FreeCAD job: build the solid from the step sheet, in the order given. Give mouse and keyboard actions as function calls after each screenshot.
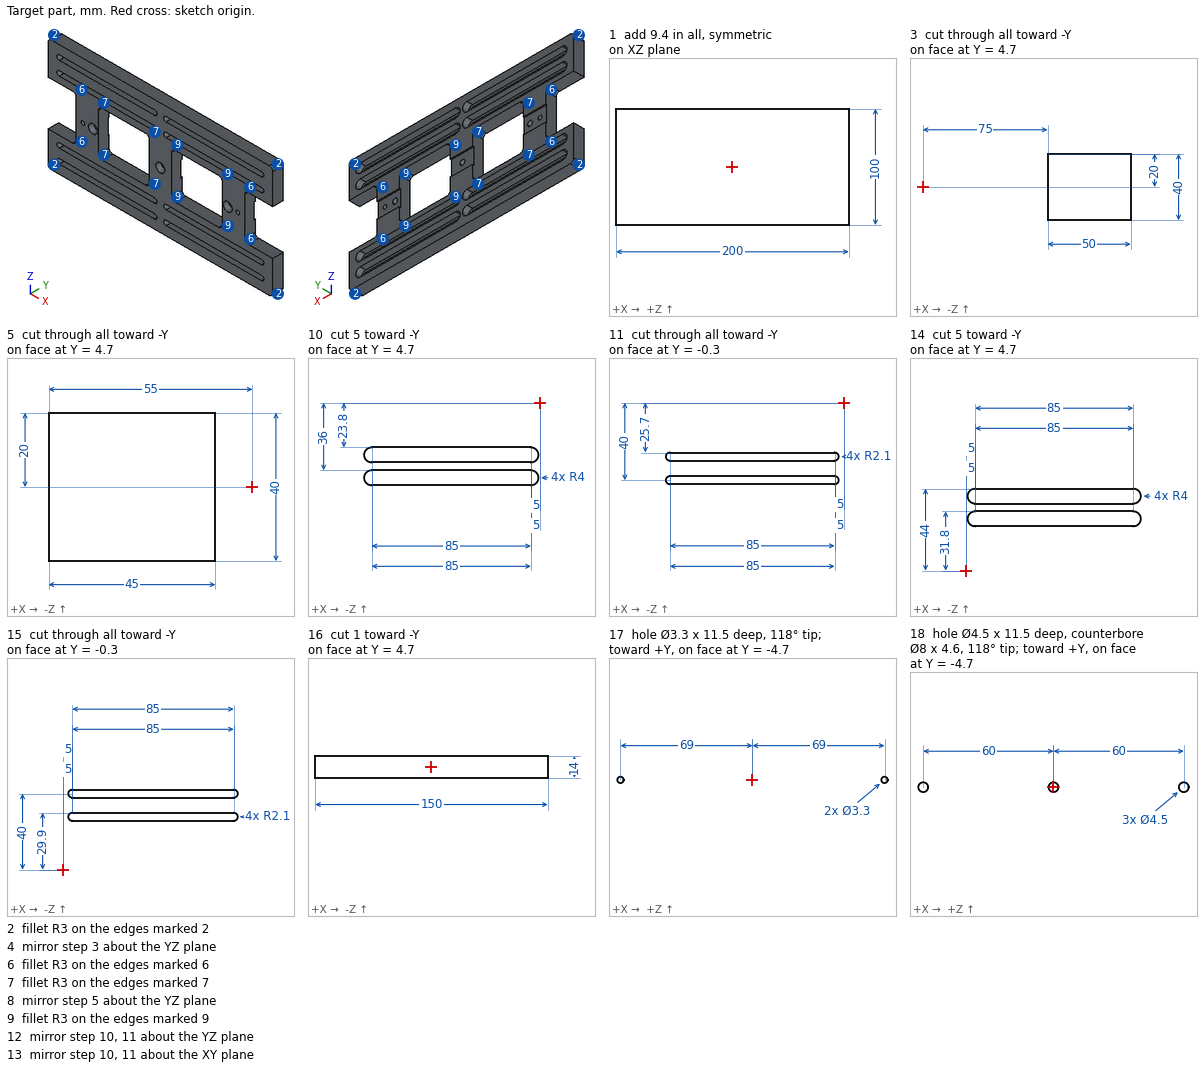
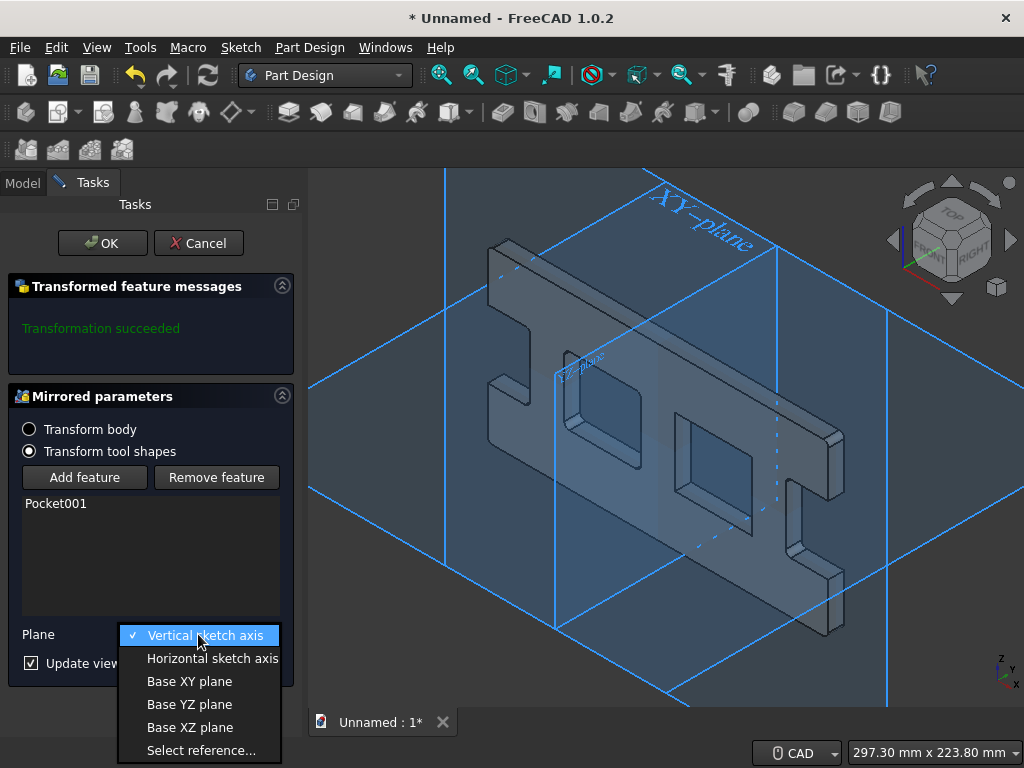
click(198, 704)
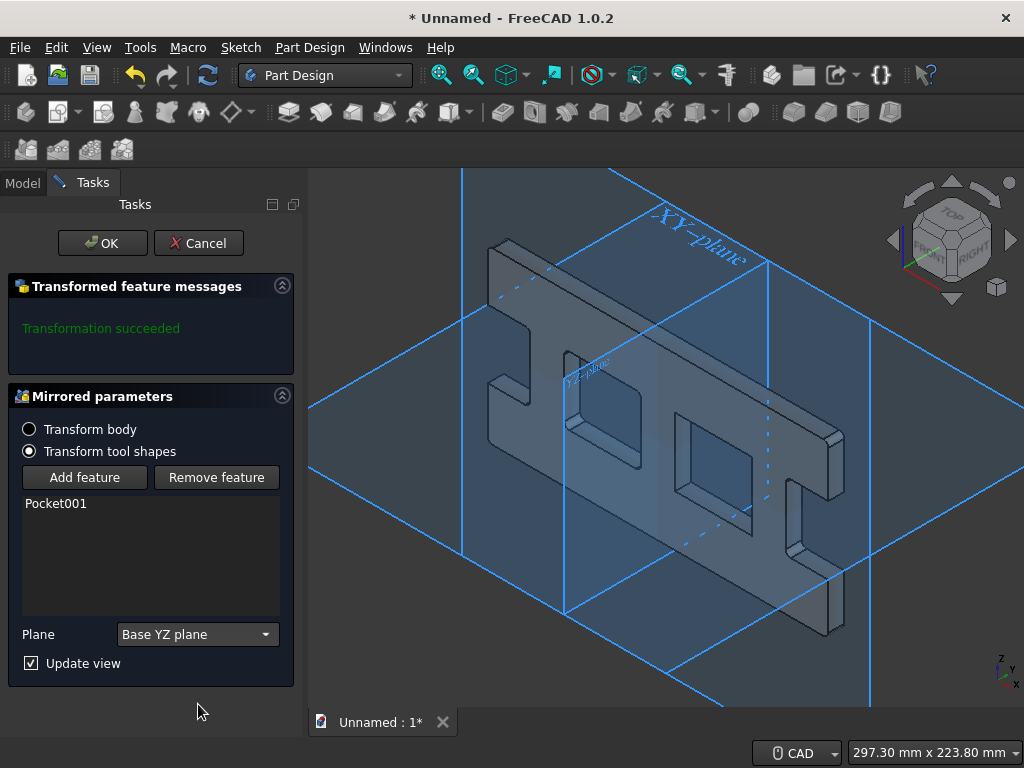
click(103, 243)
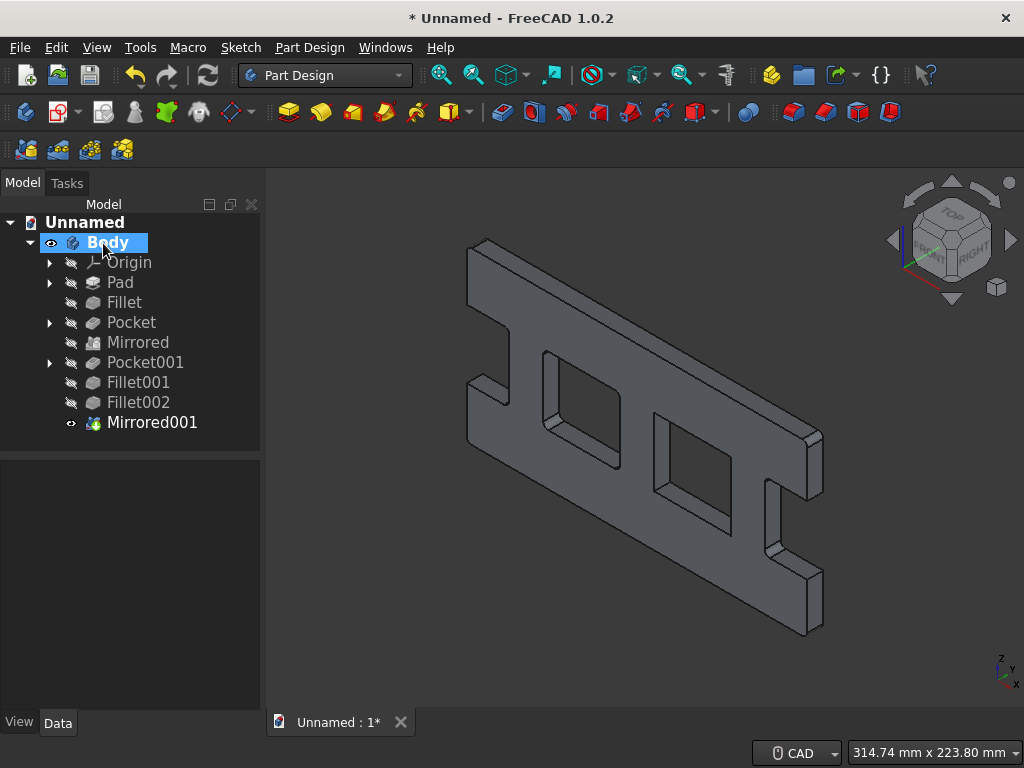
key(2)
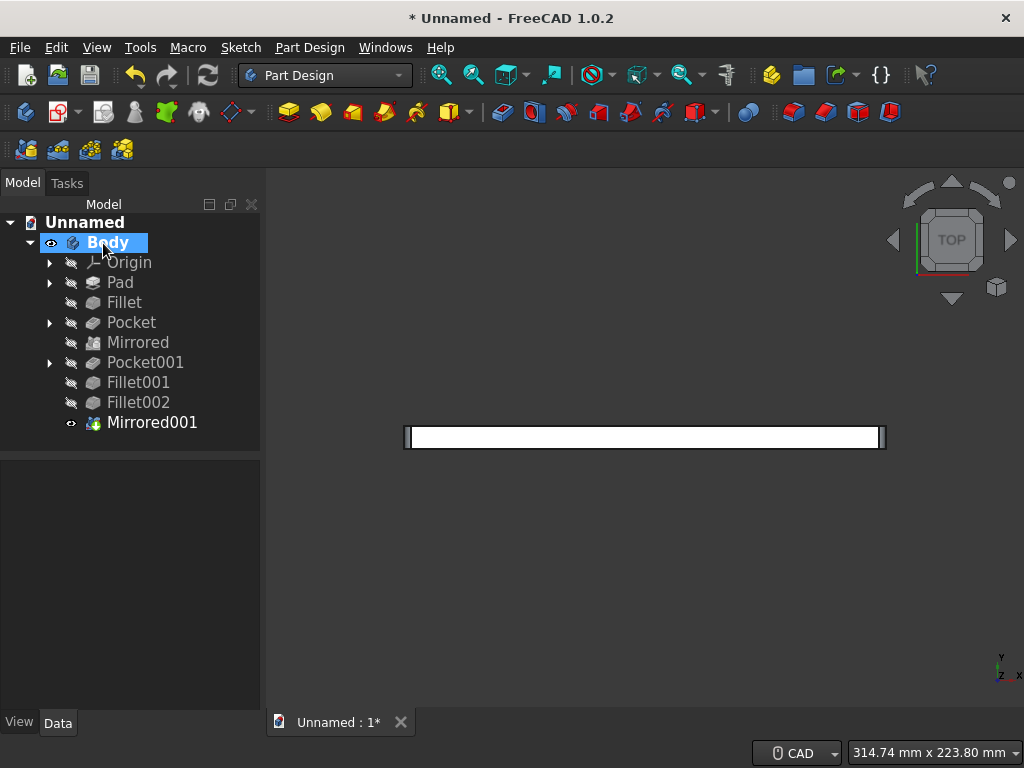
key(0)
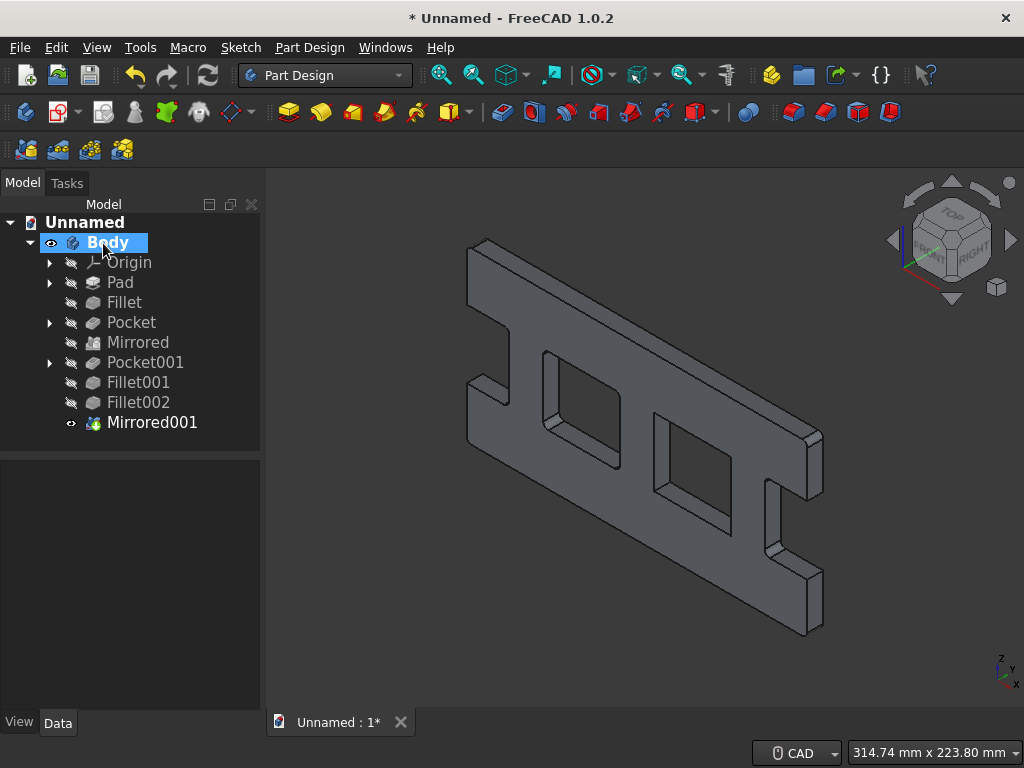
key(1)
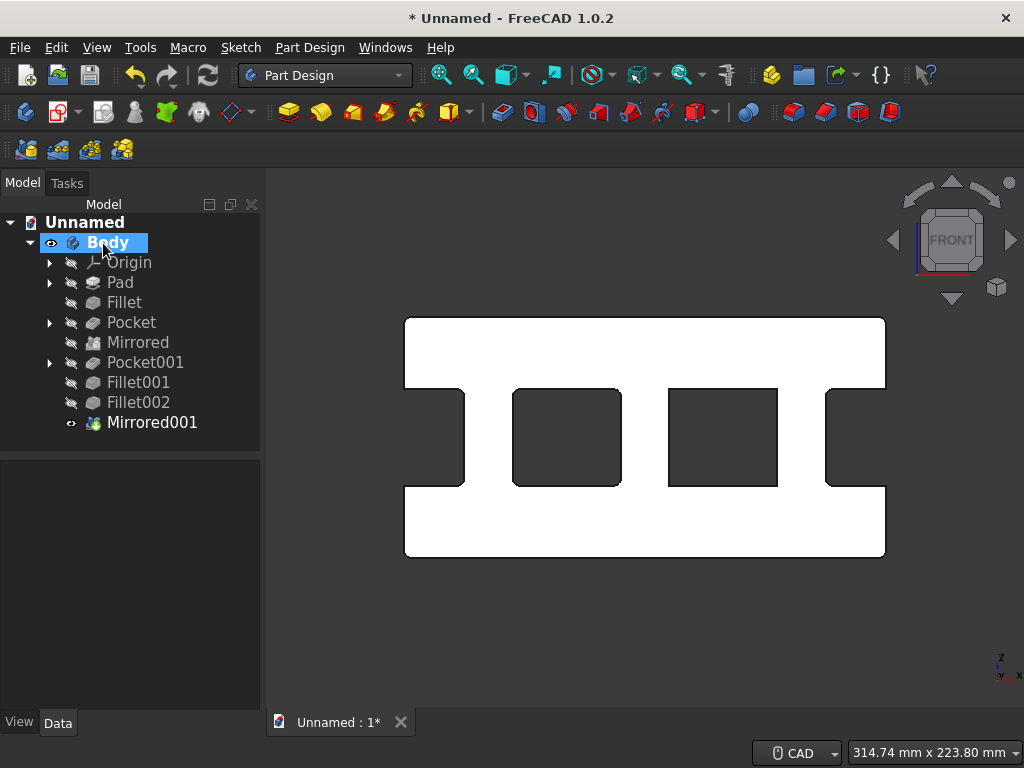
key(3)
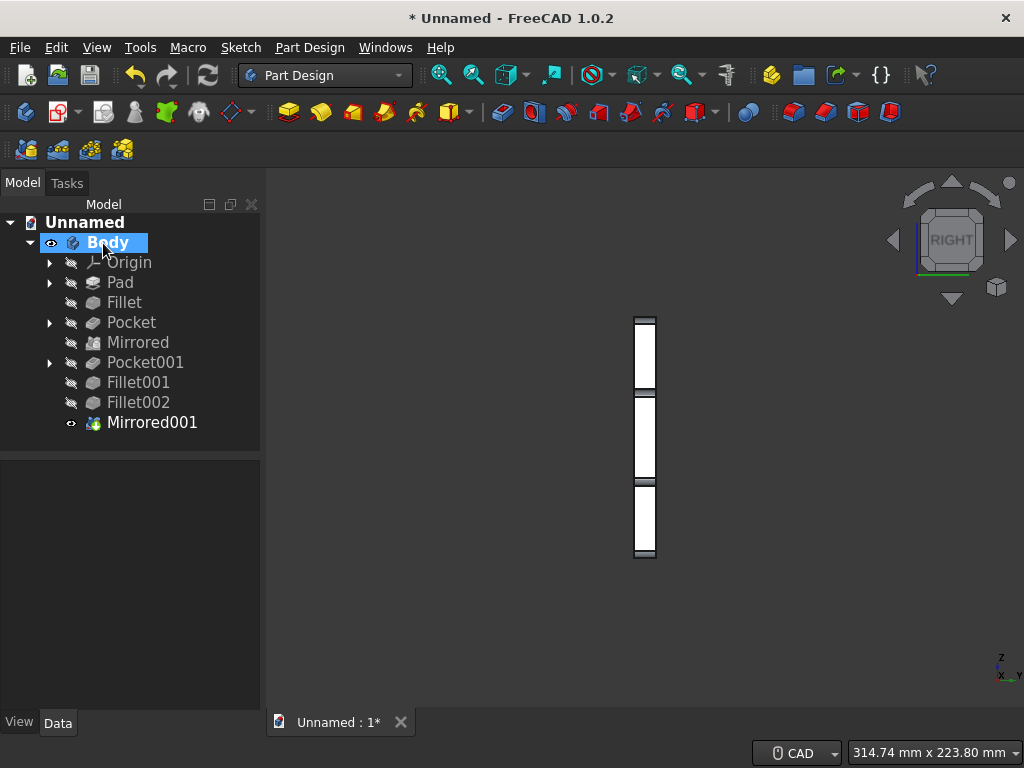
key(v)
key(f)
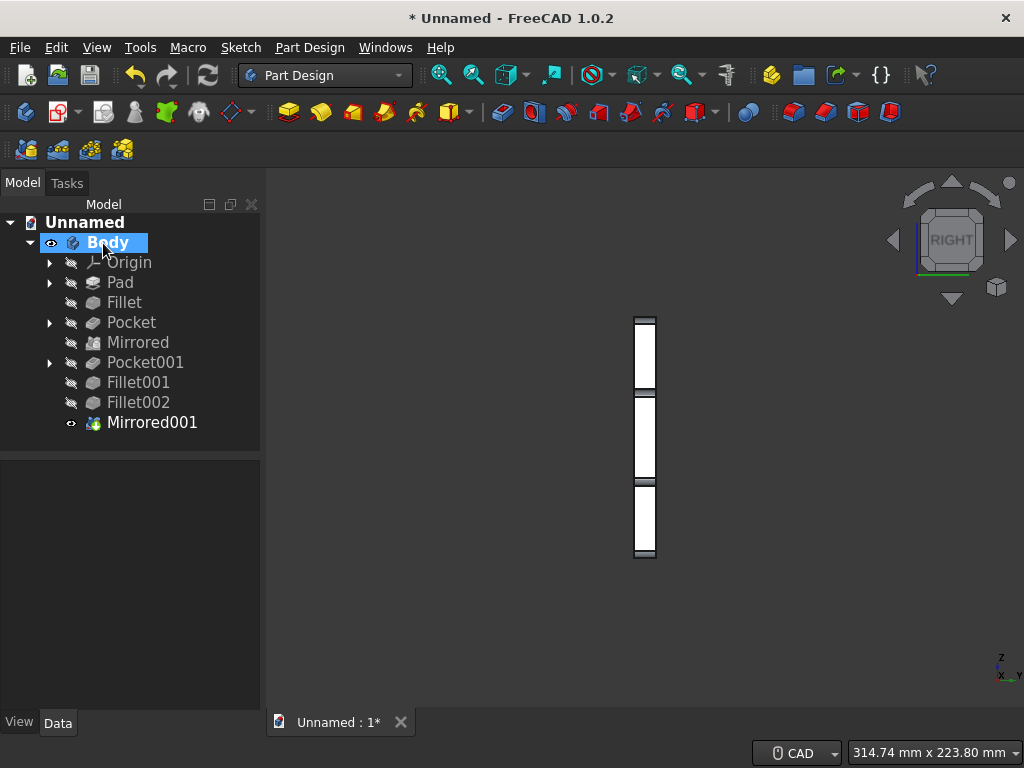
key(5)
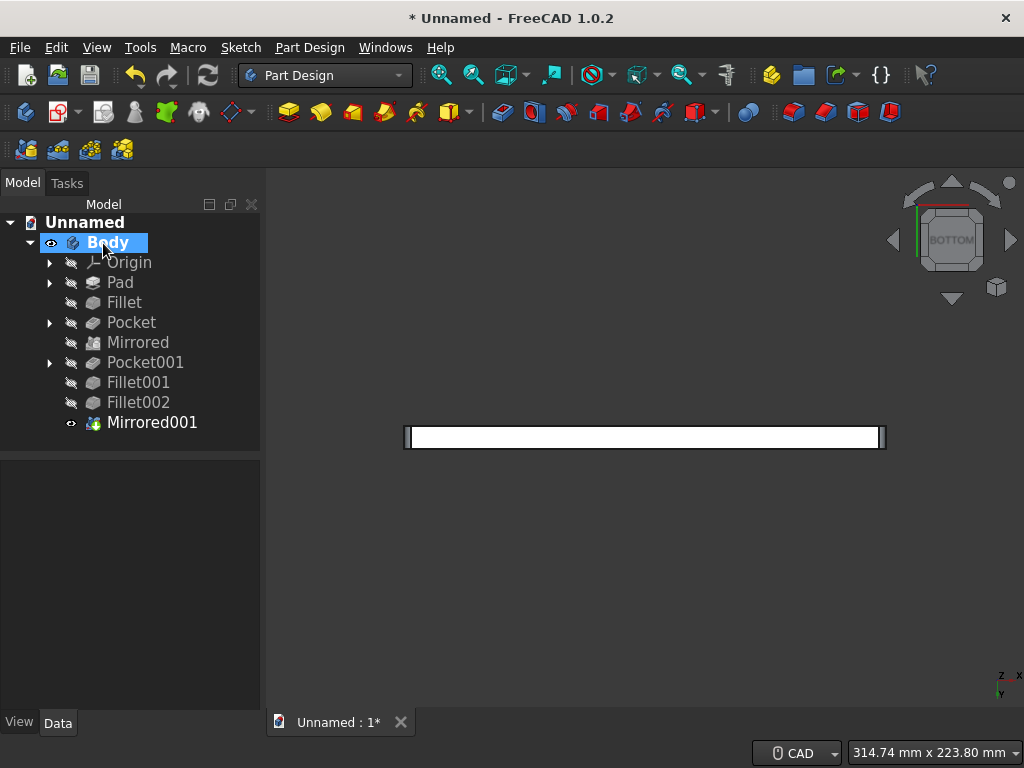
key(4)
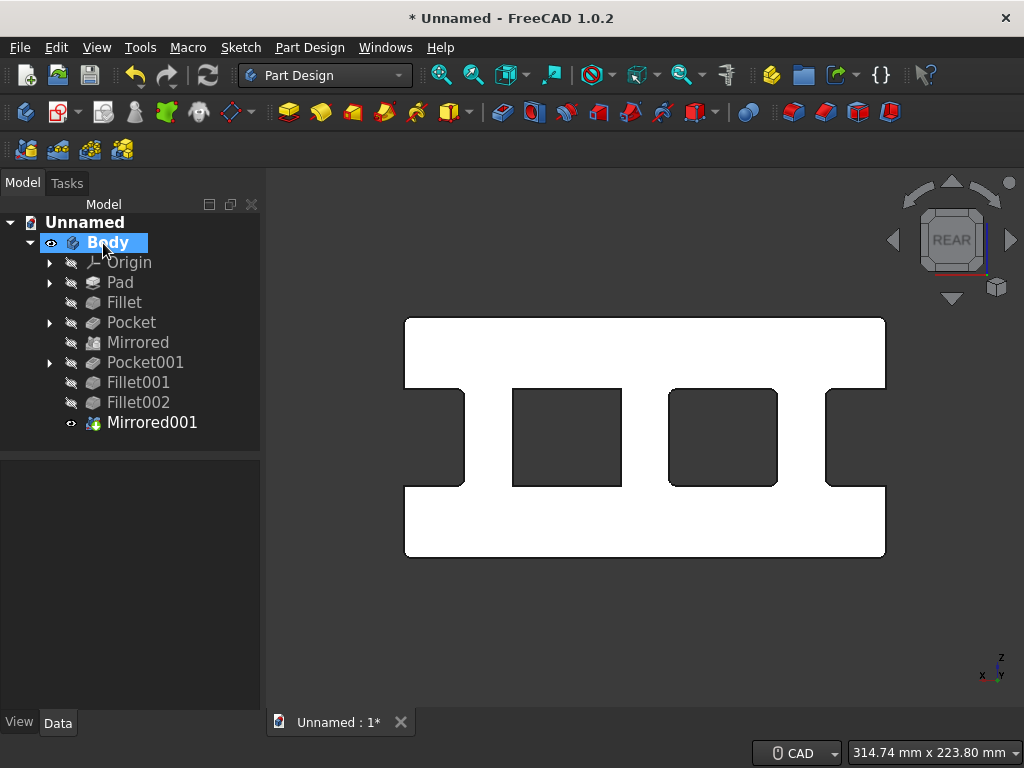
key(6)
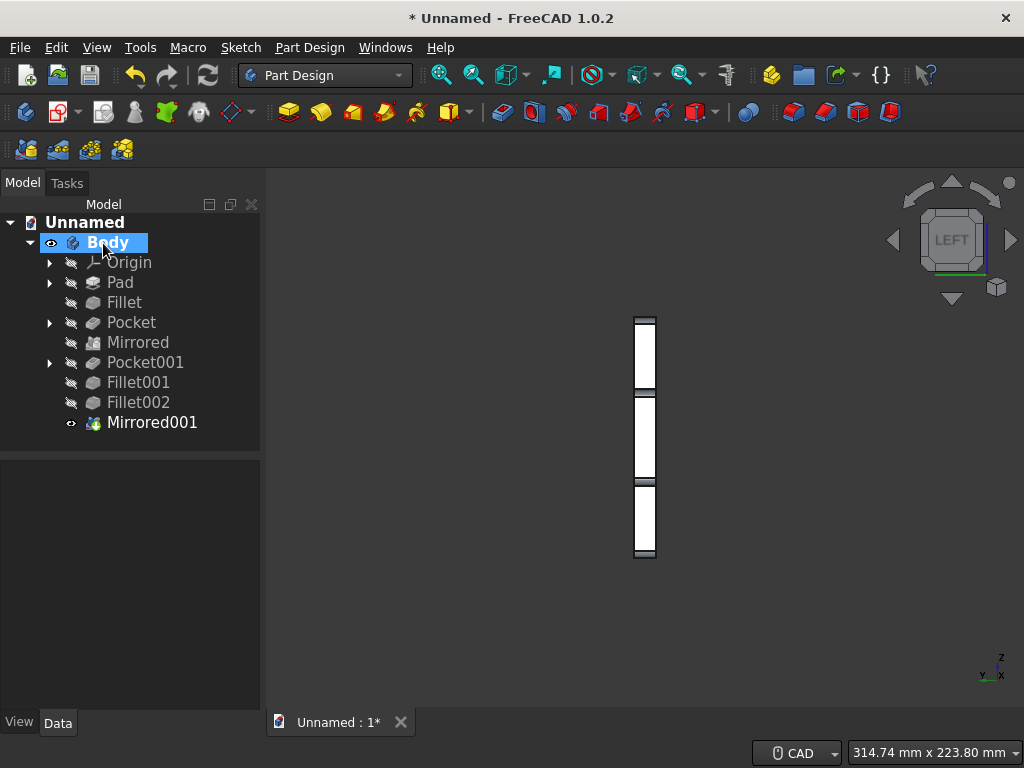
key(v)
key(f)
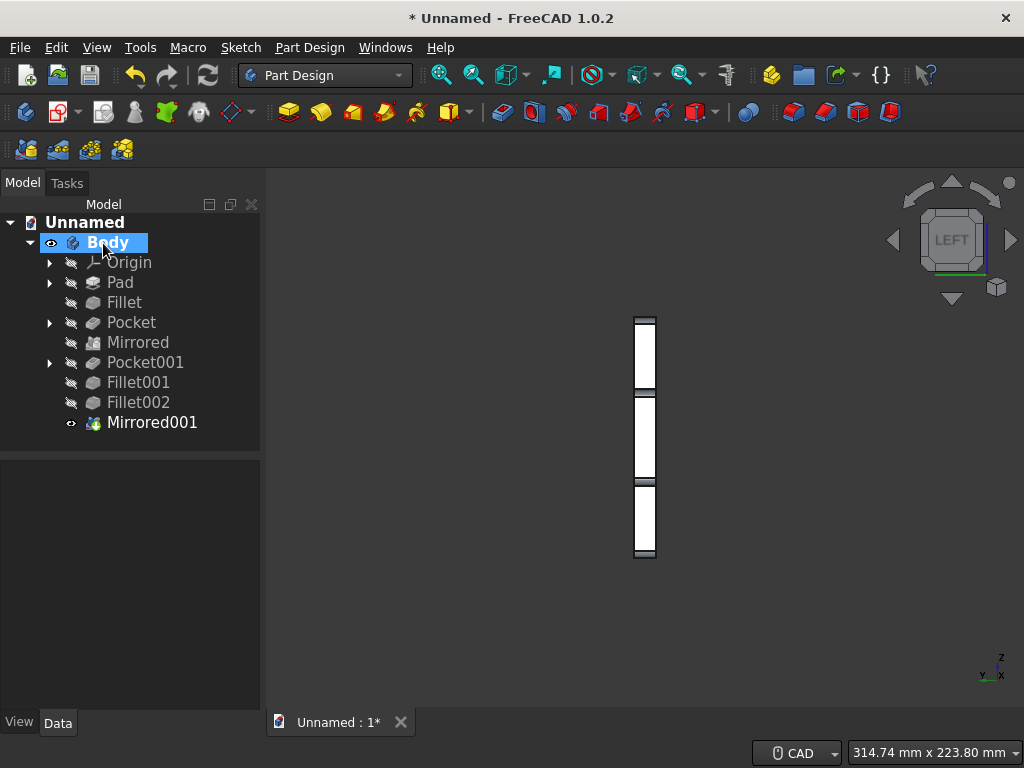
key(v)
key(3)